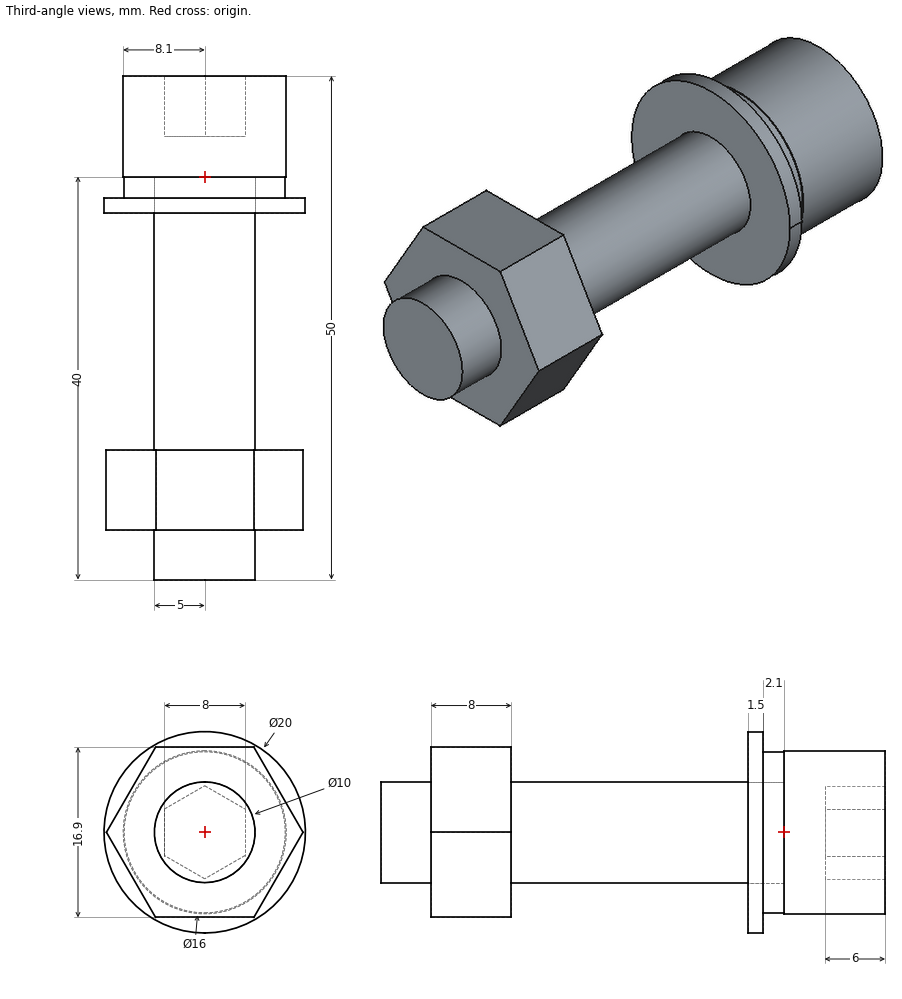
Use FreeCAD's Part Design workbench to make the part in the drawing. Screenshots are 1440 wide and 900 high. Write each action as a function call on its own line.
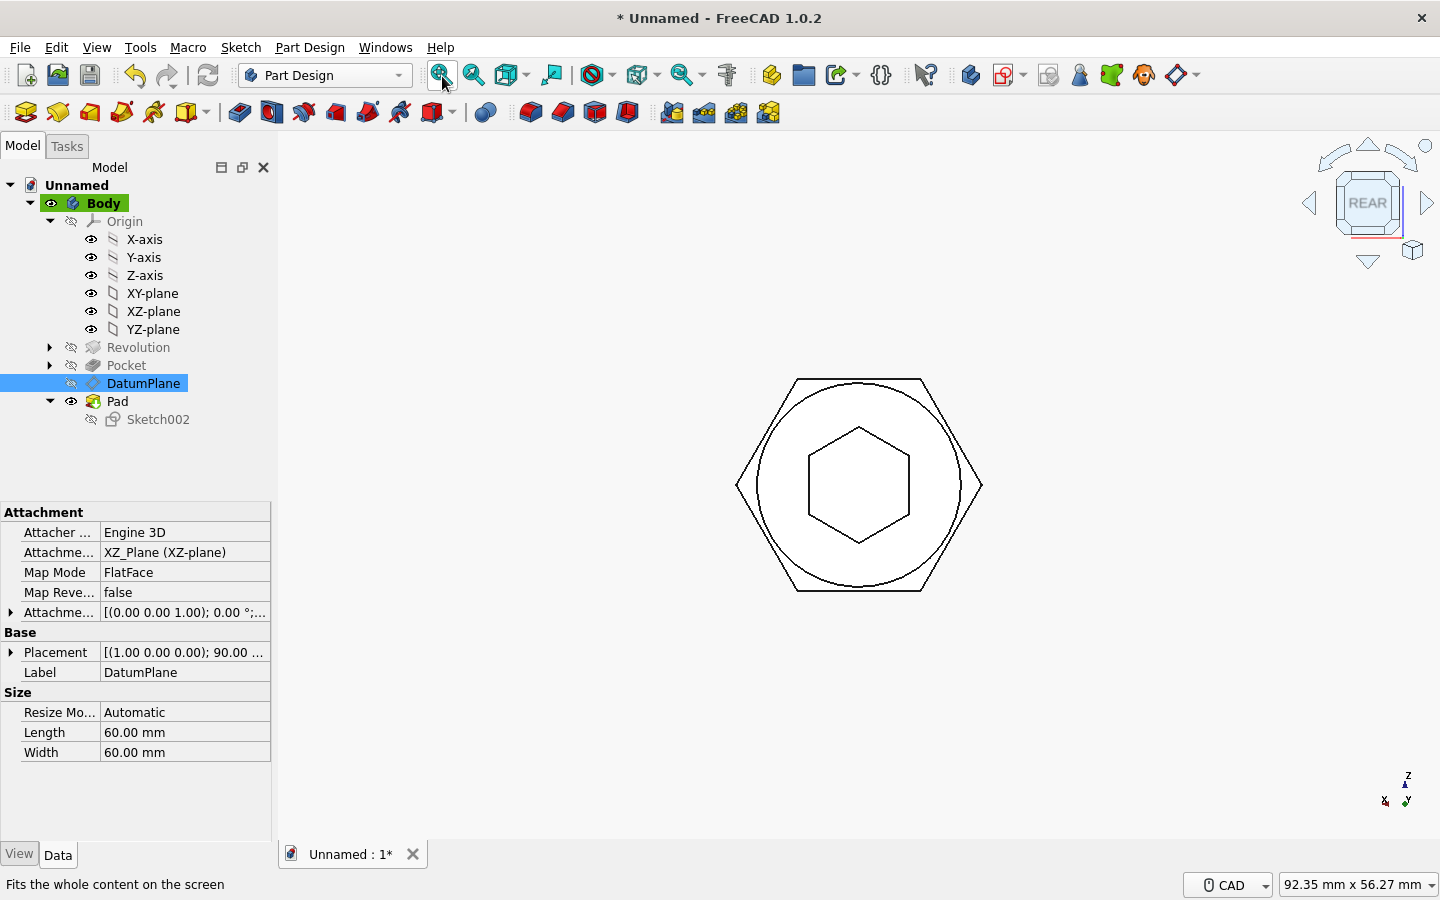
click(318, 799)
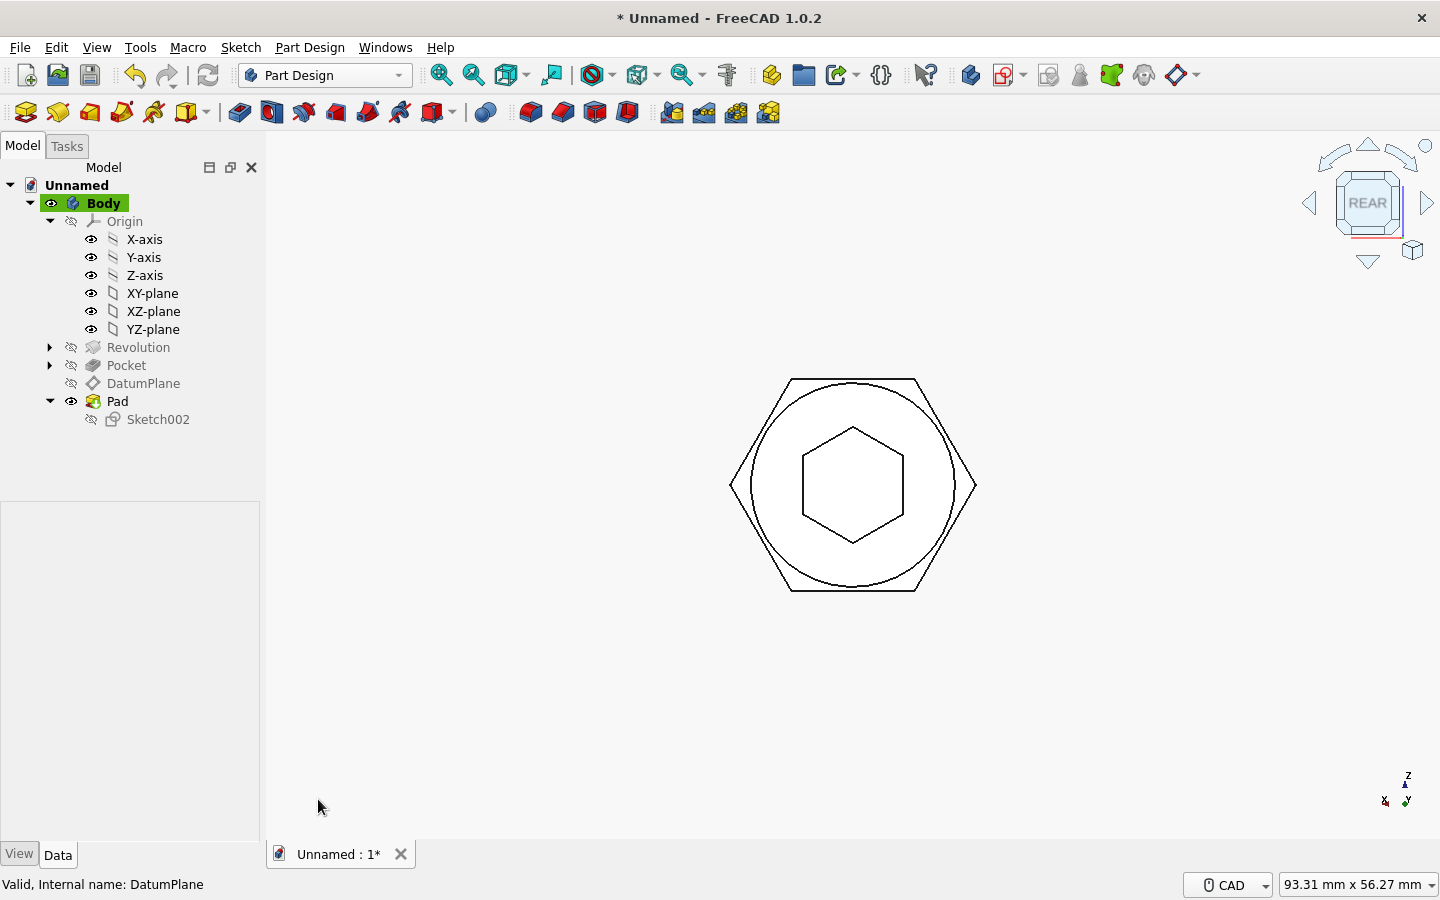
click(972, 76)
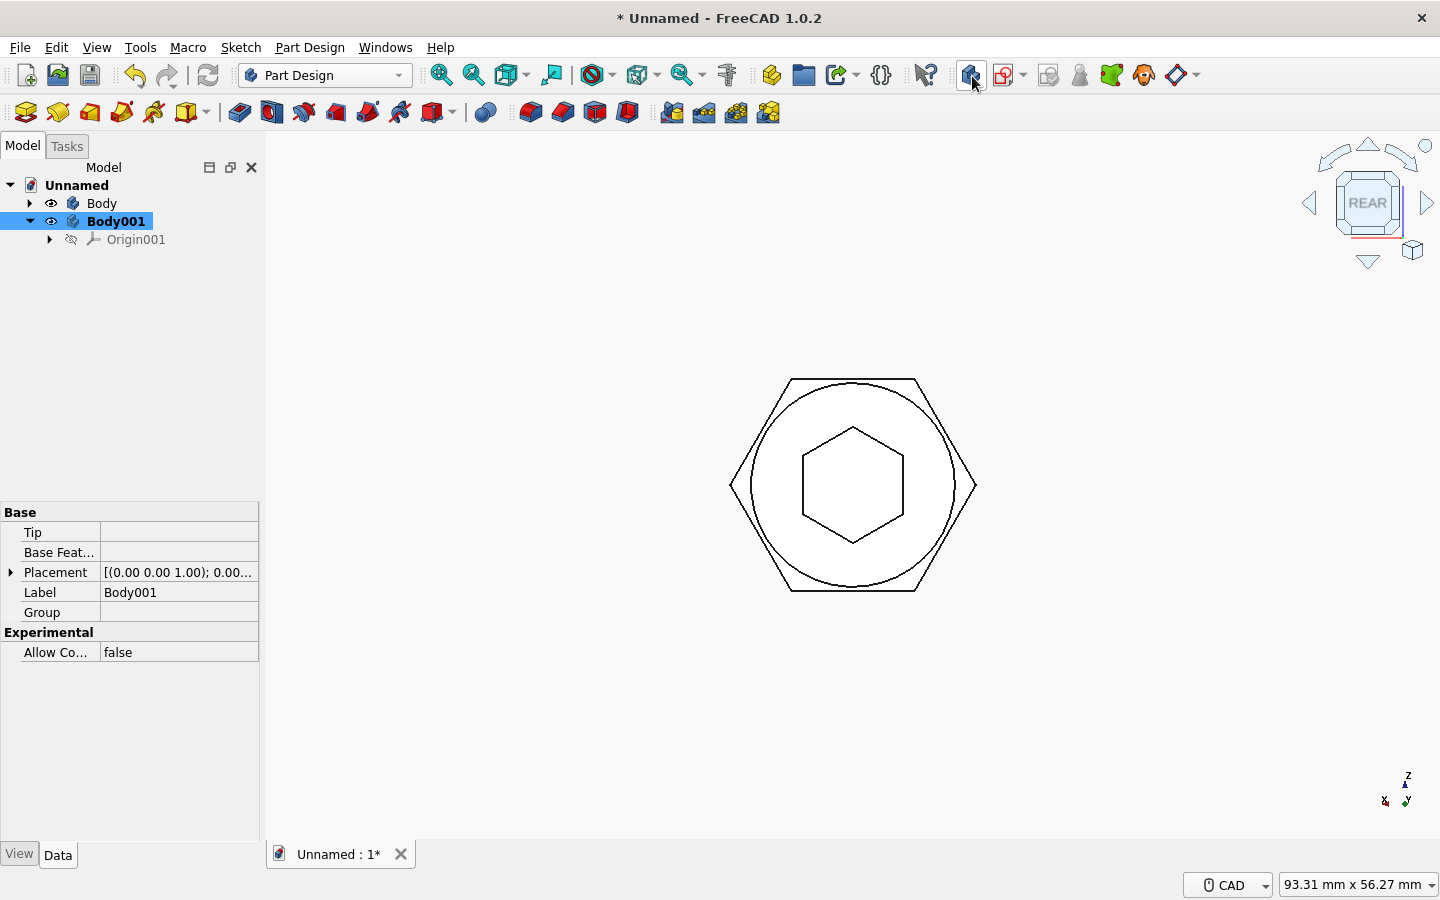
click(306, 799)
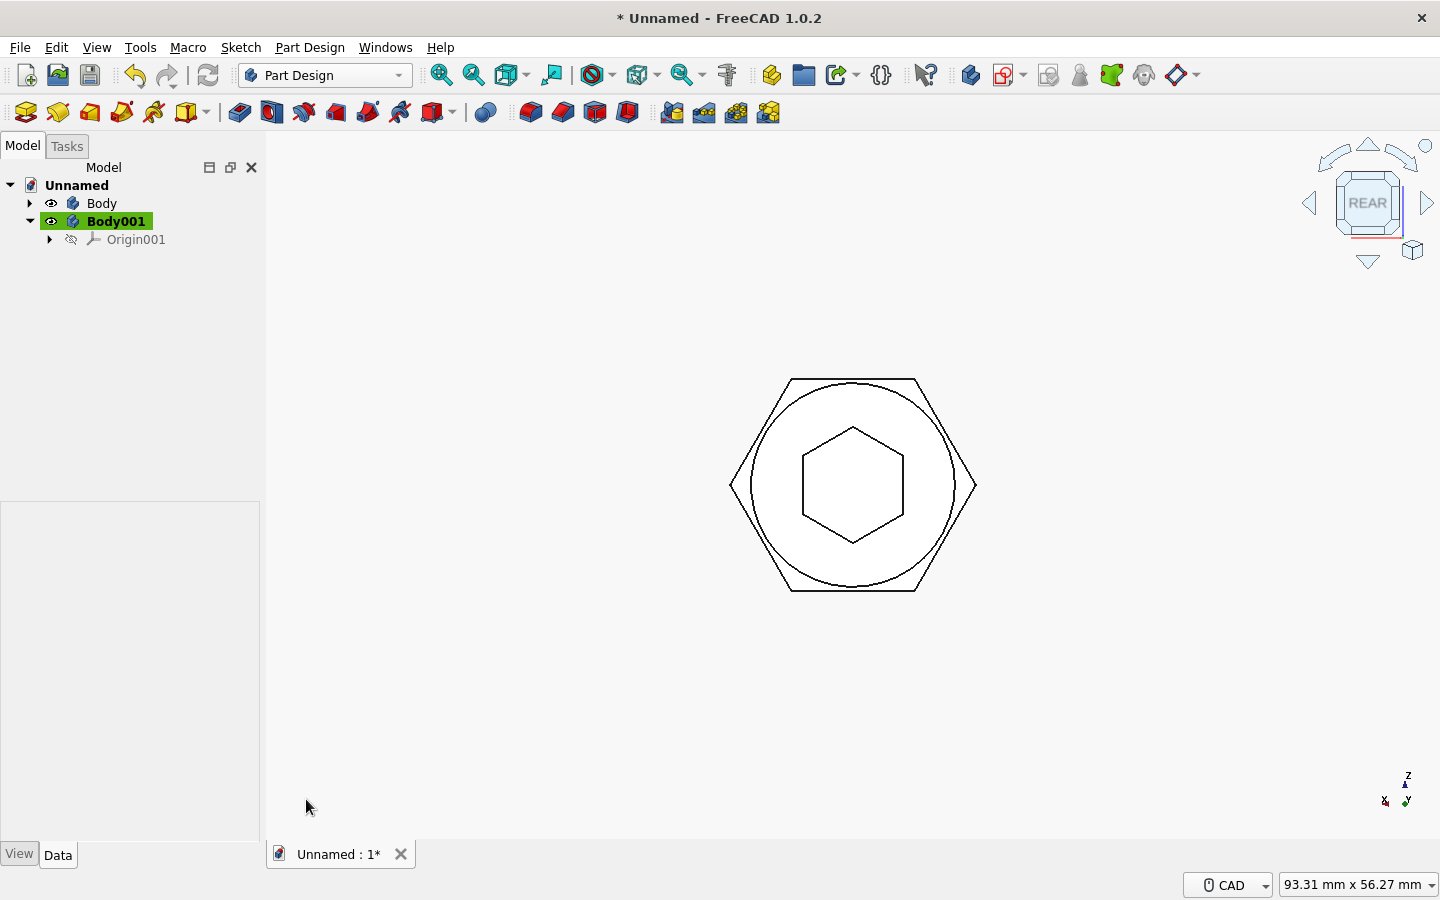
click(1004, 76)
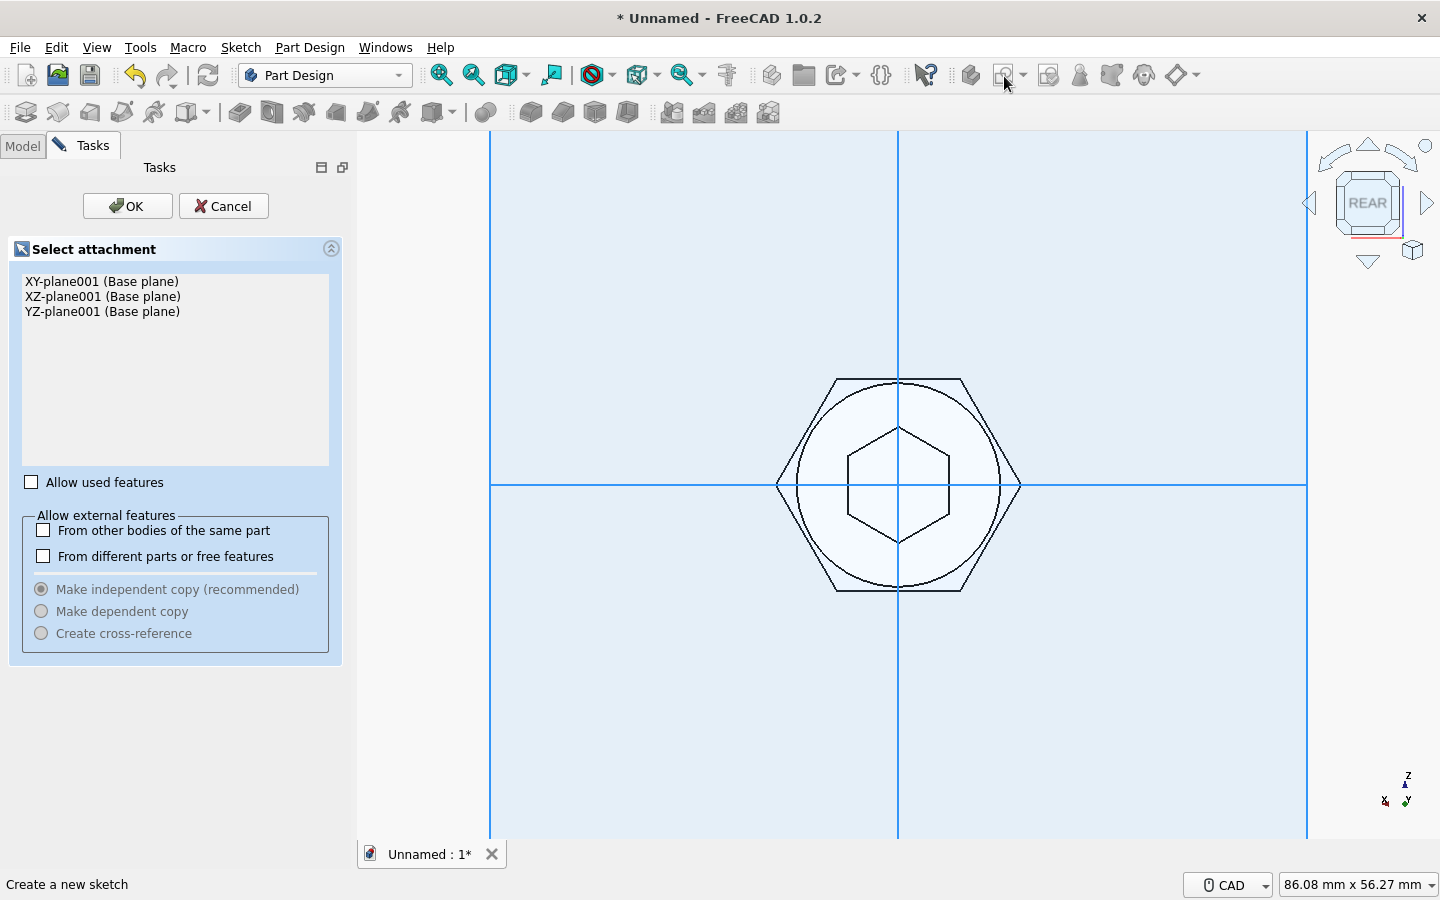
click(82, 296)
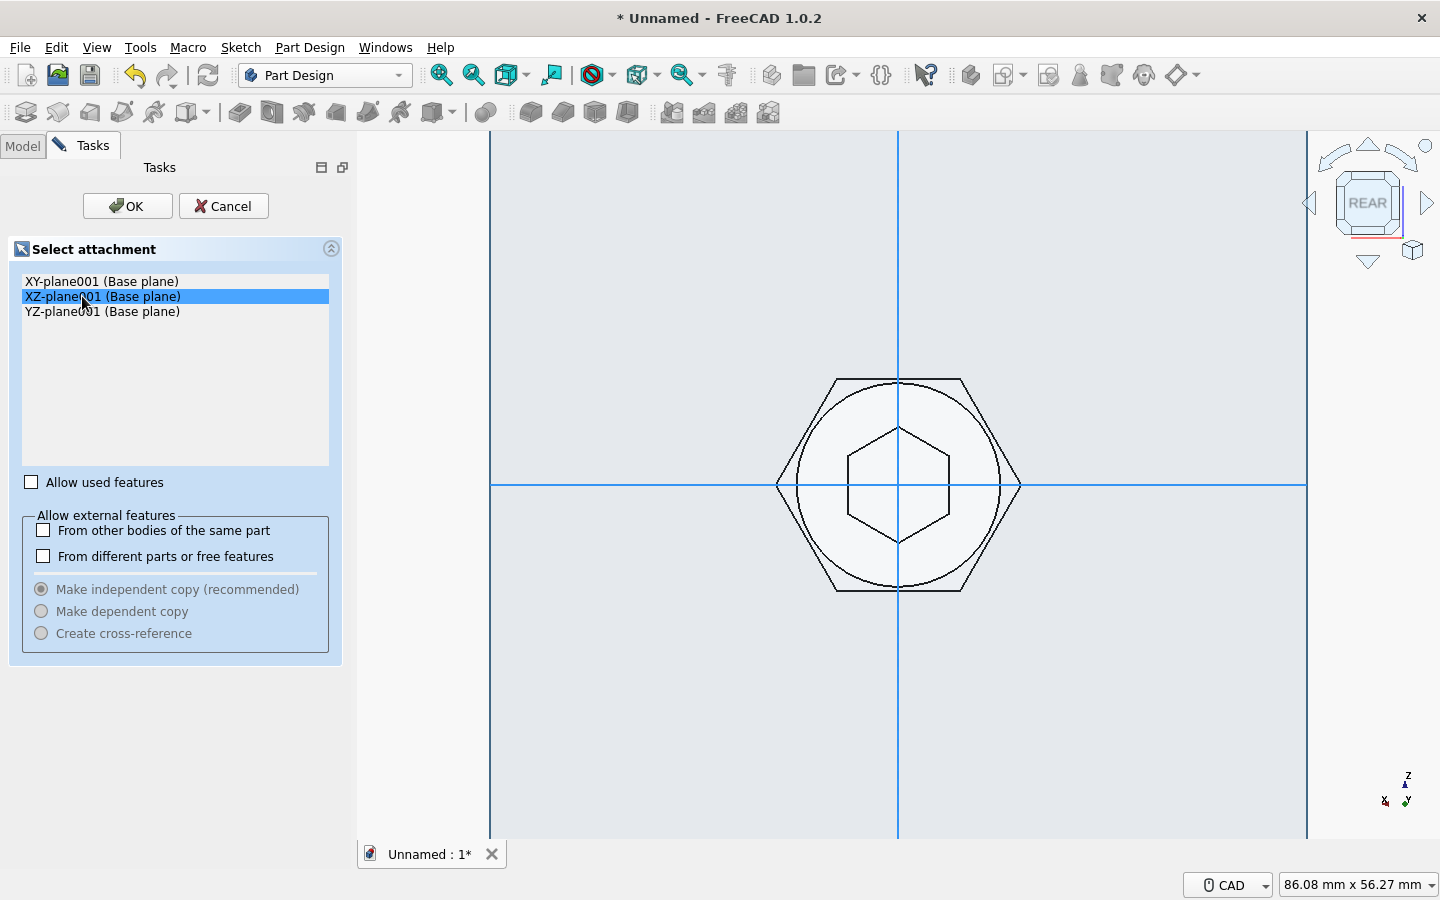
click(128, 206)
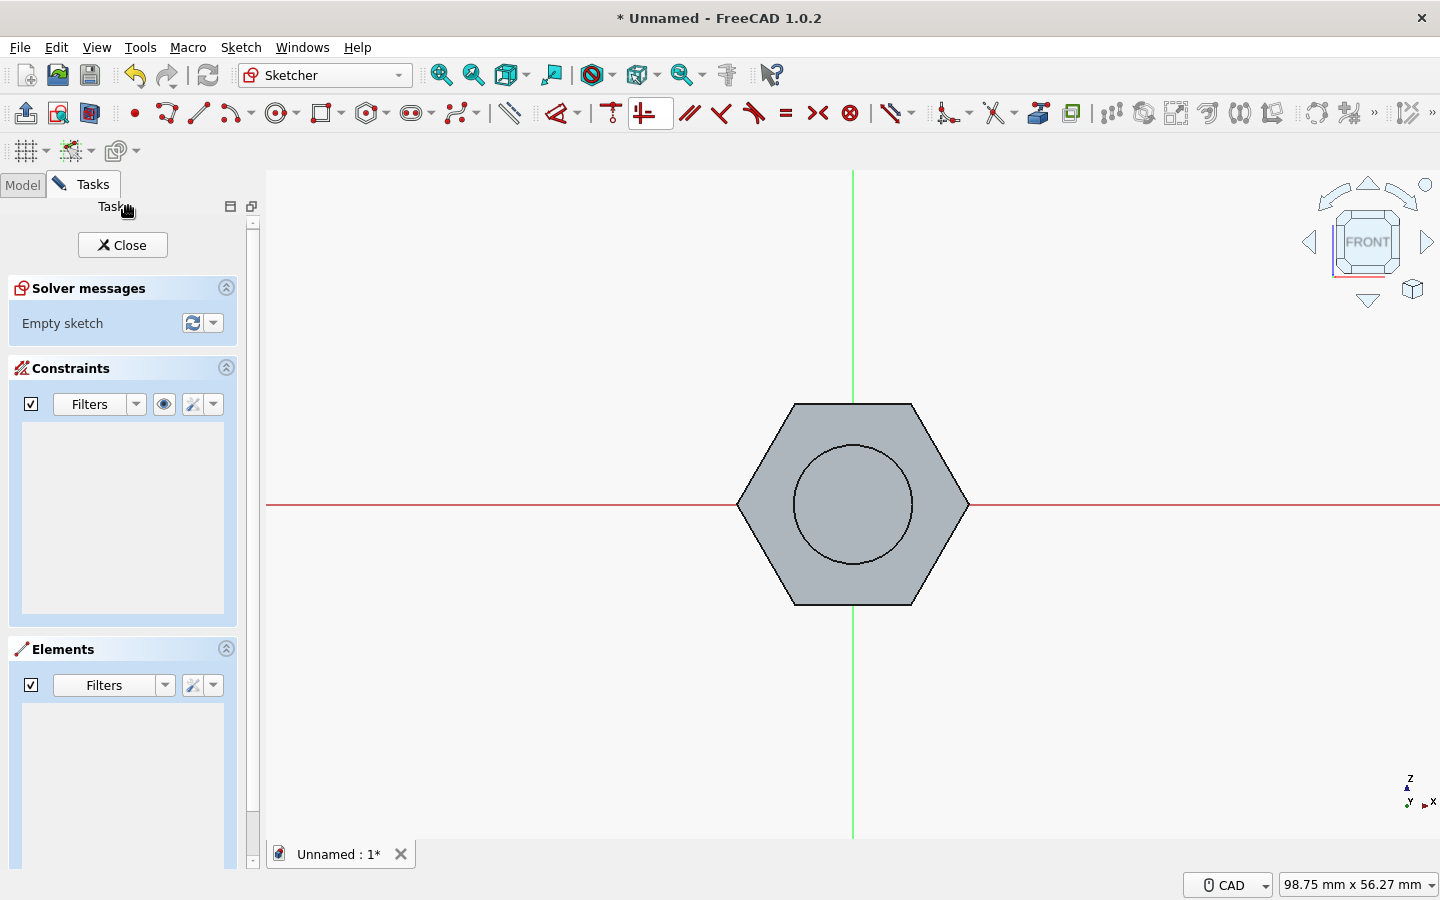
scroll(909, 504, up, 4)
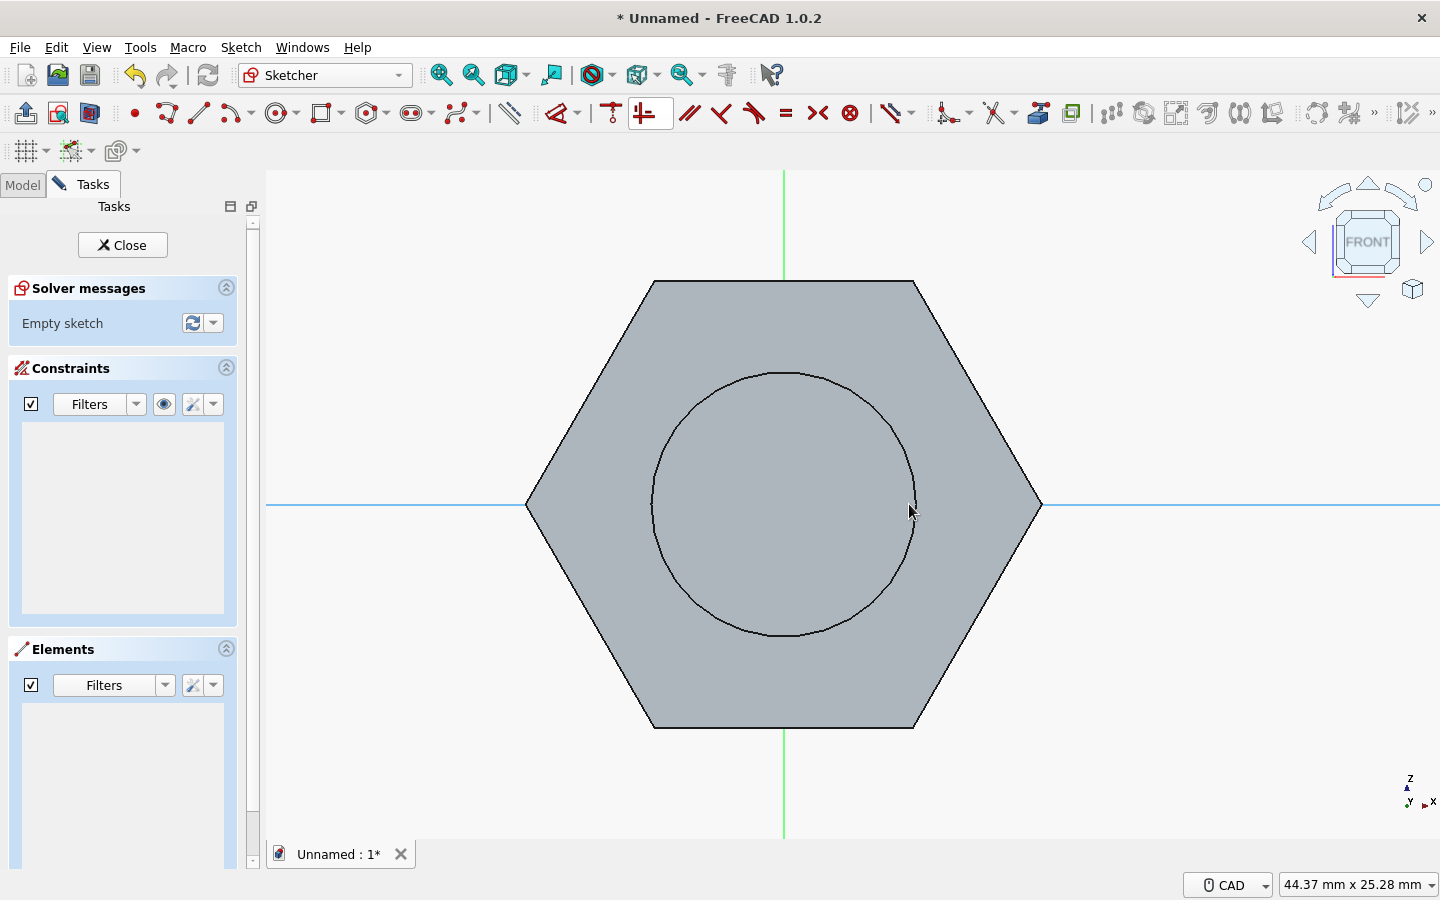
click(276, 114)